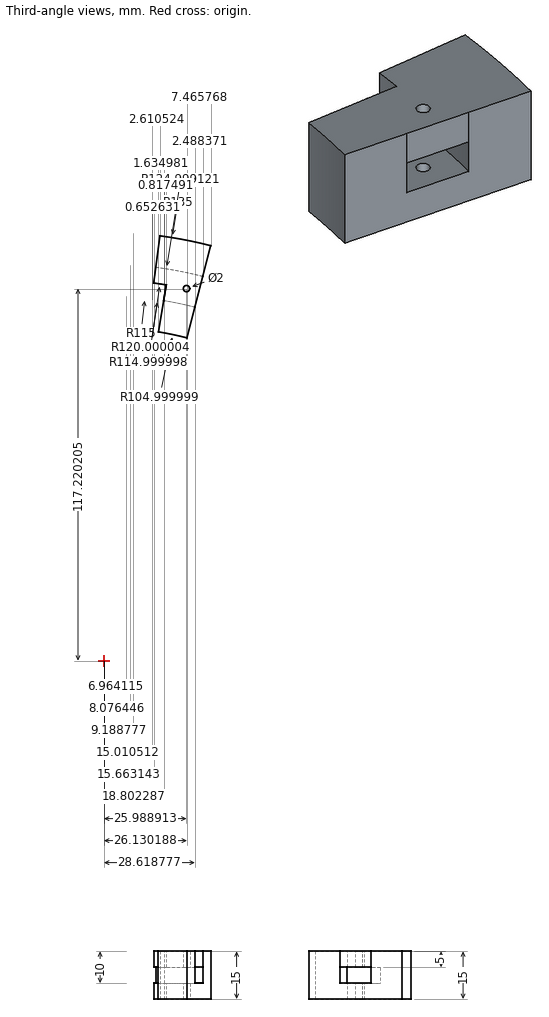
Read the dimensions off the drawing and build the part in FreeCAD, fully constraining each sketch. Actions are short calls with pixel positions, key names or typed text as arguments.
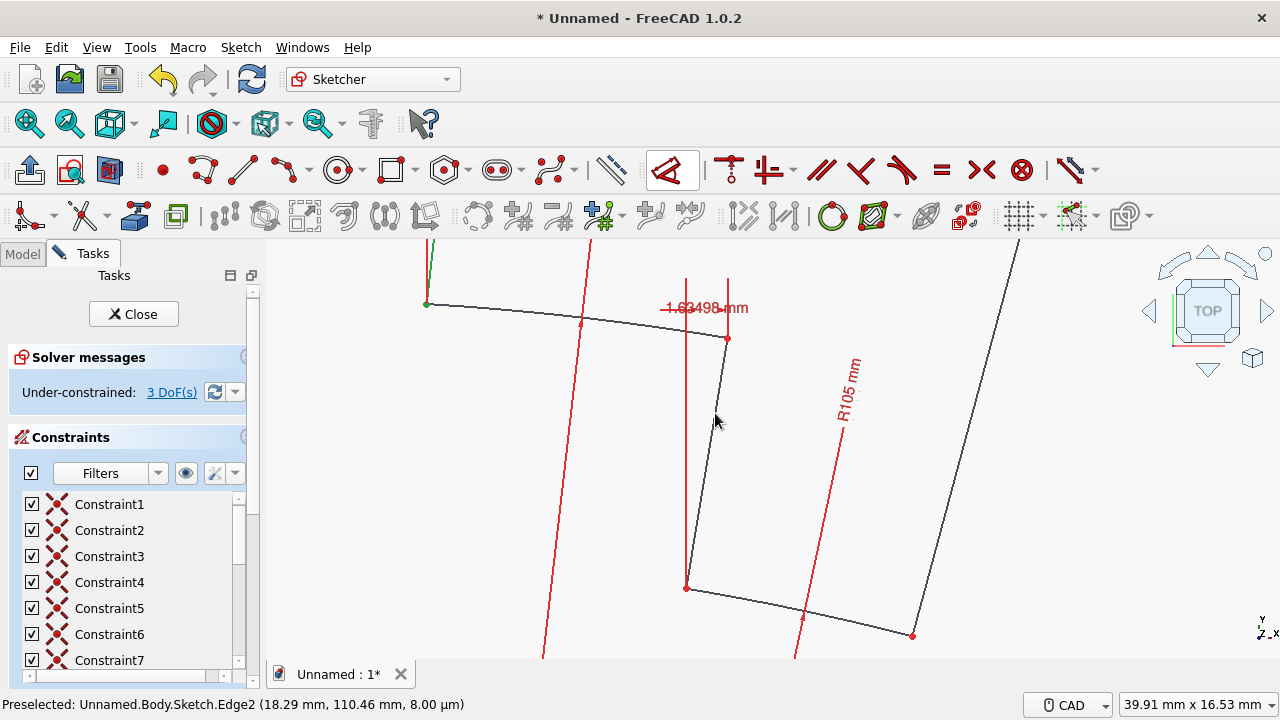
click(972, 416)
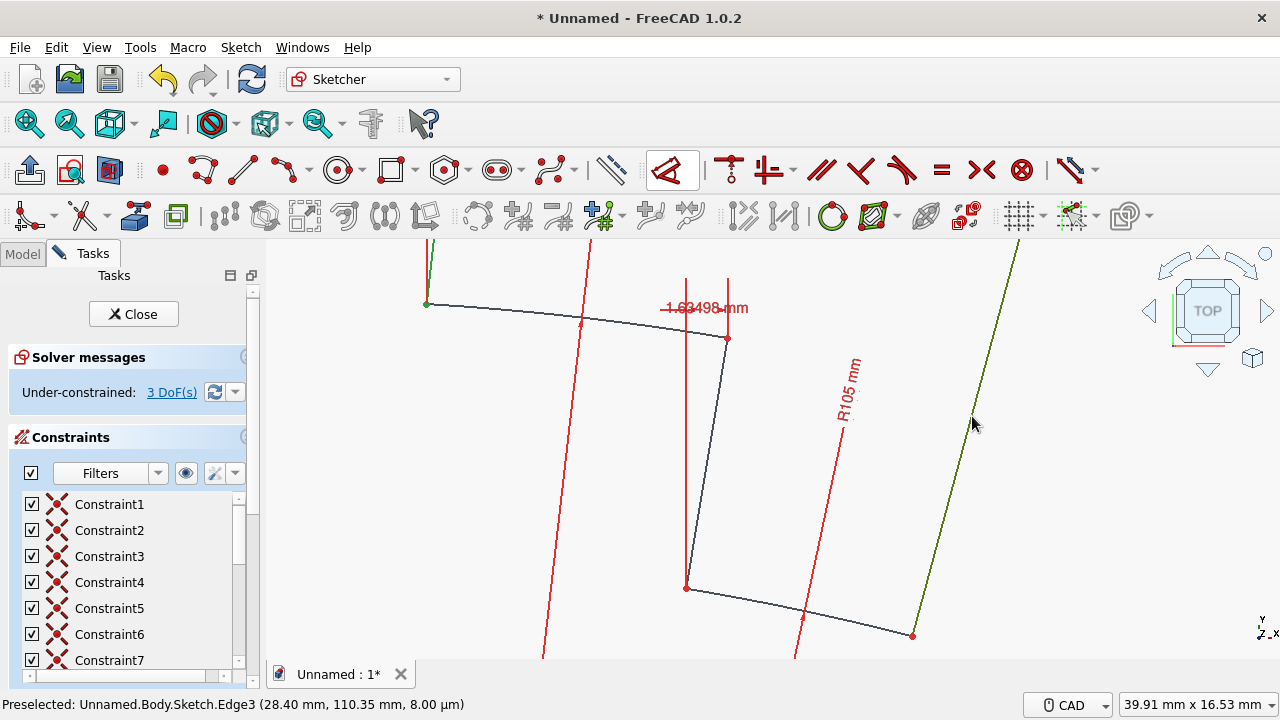
key(l)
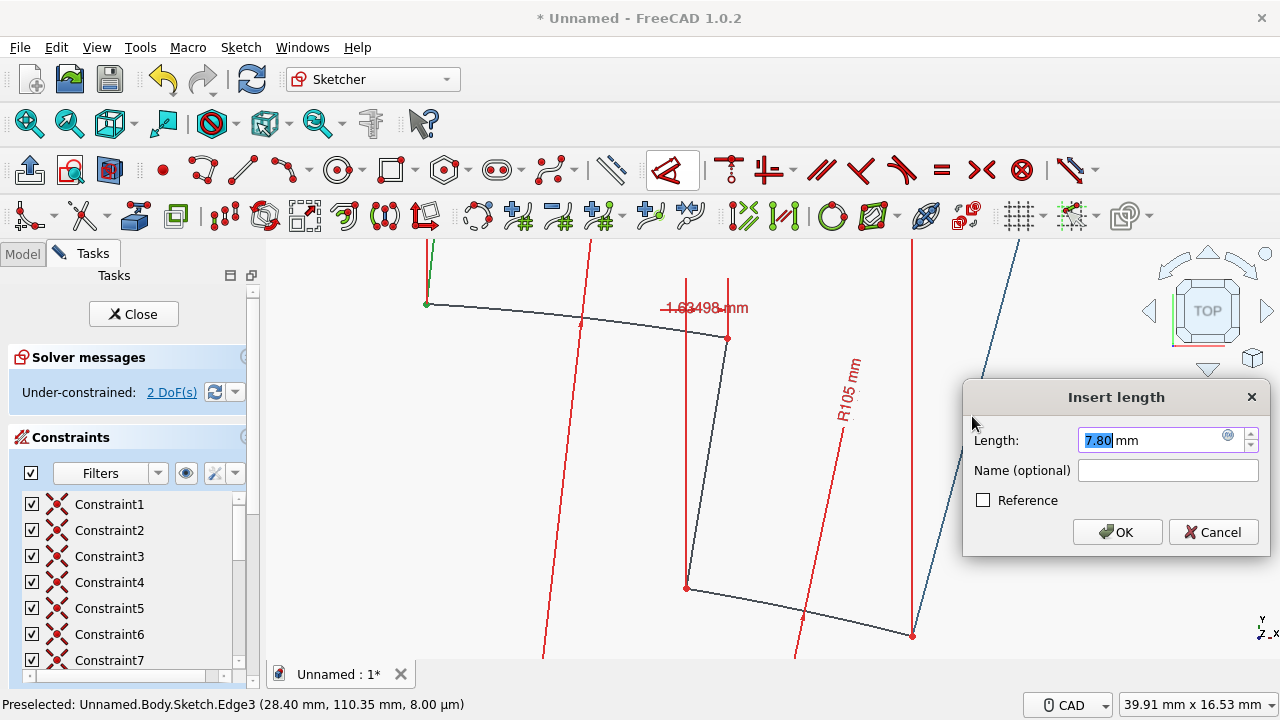
text(7.465768)
key(Return)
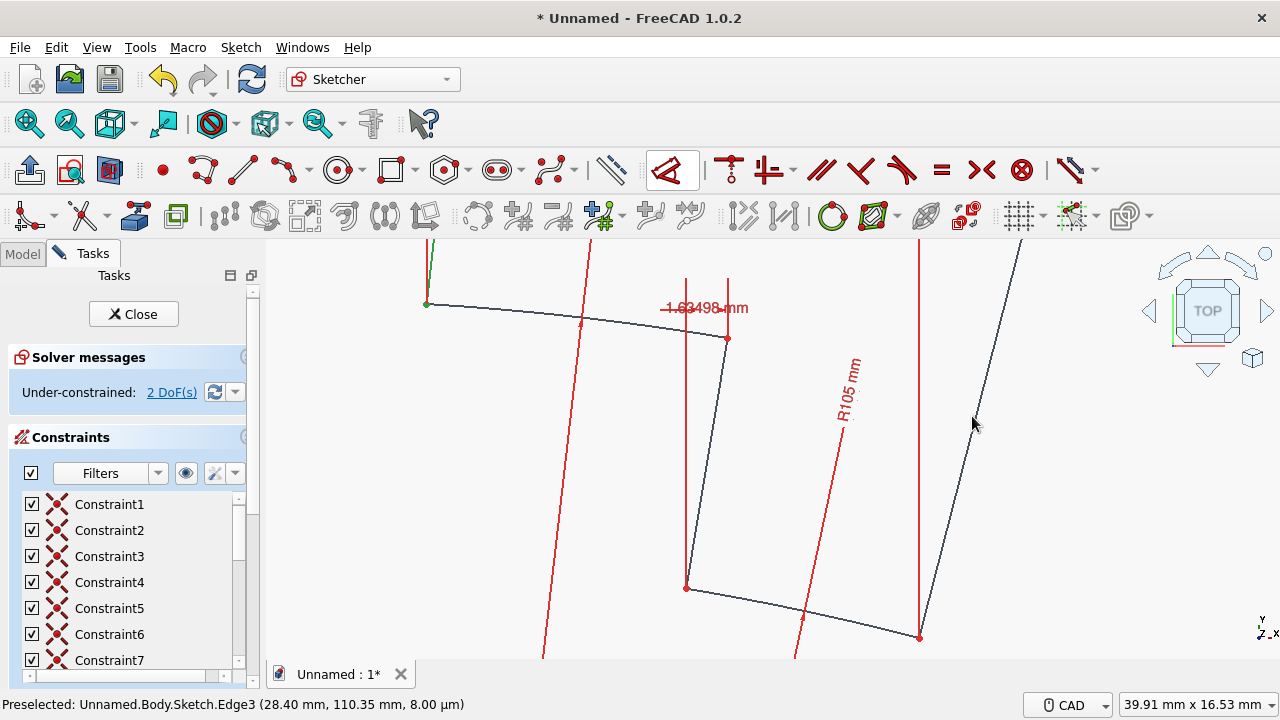
click(728, 338)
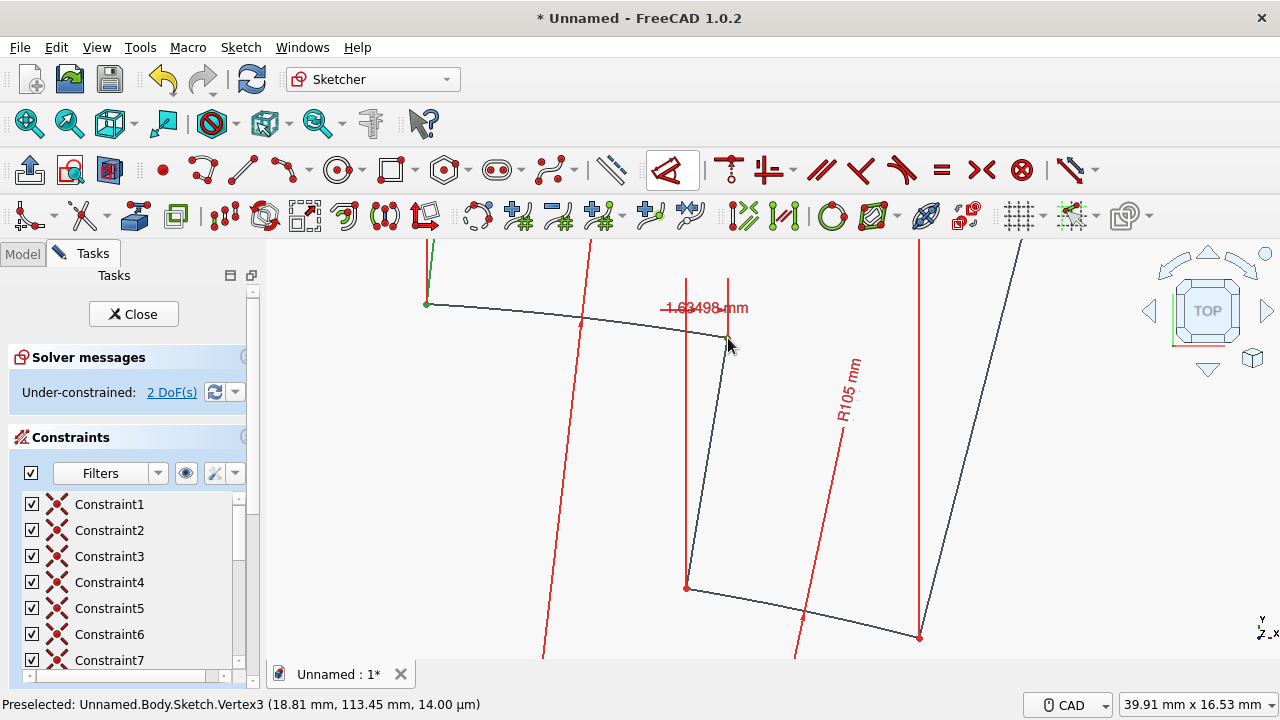
click(694, 170)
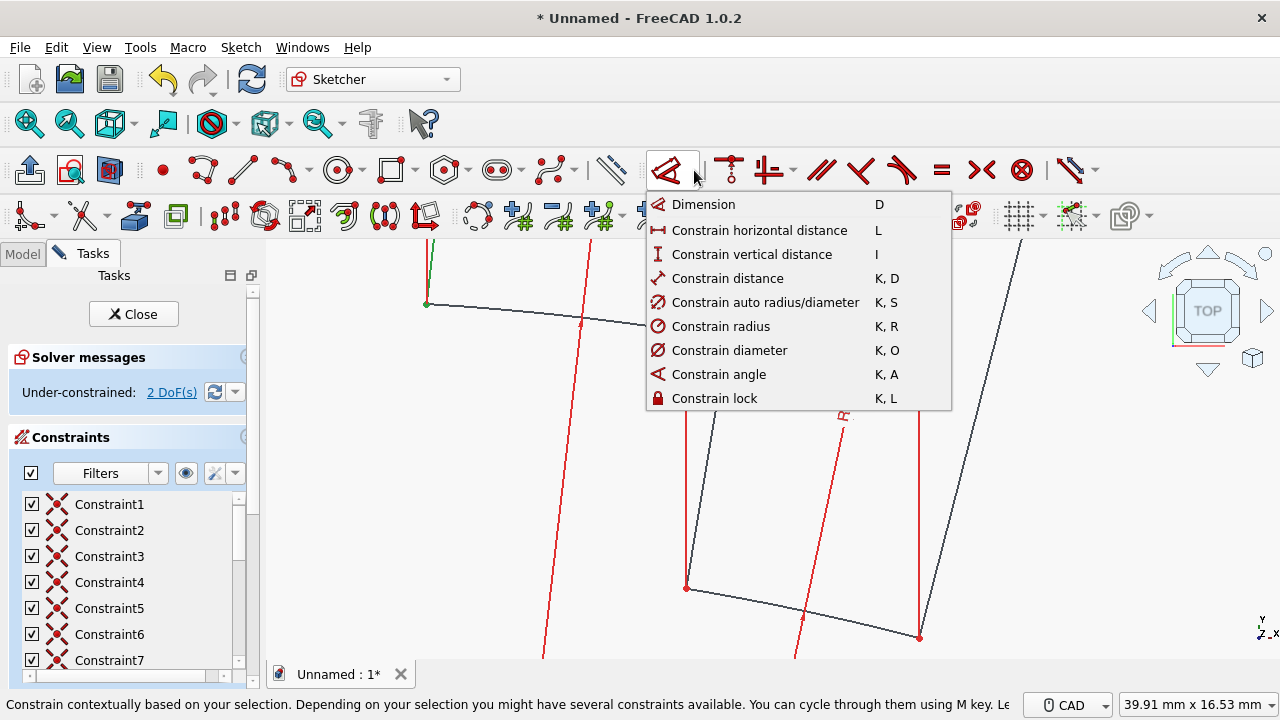
click(799, 230)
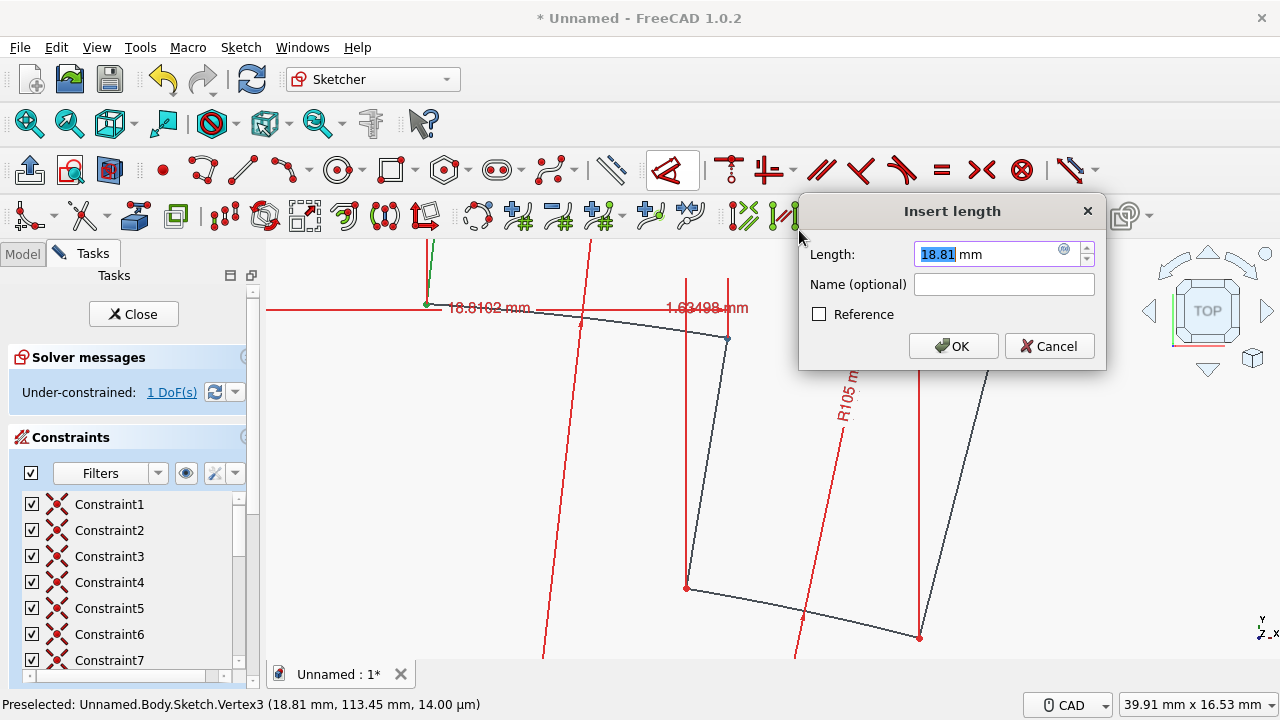
text(18.802287)
key(Return)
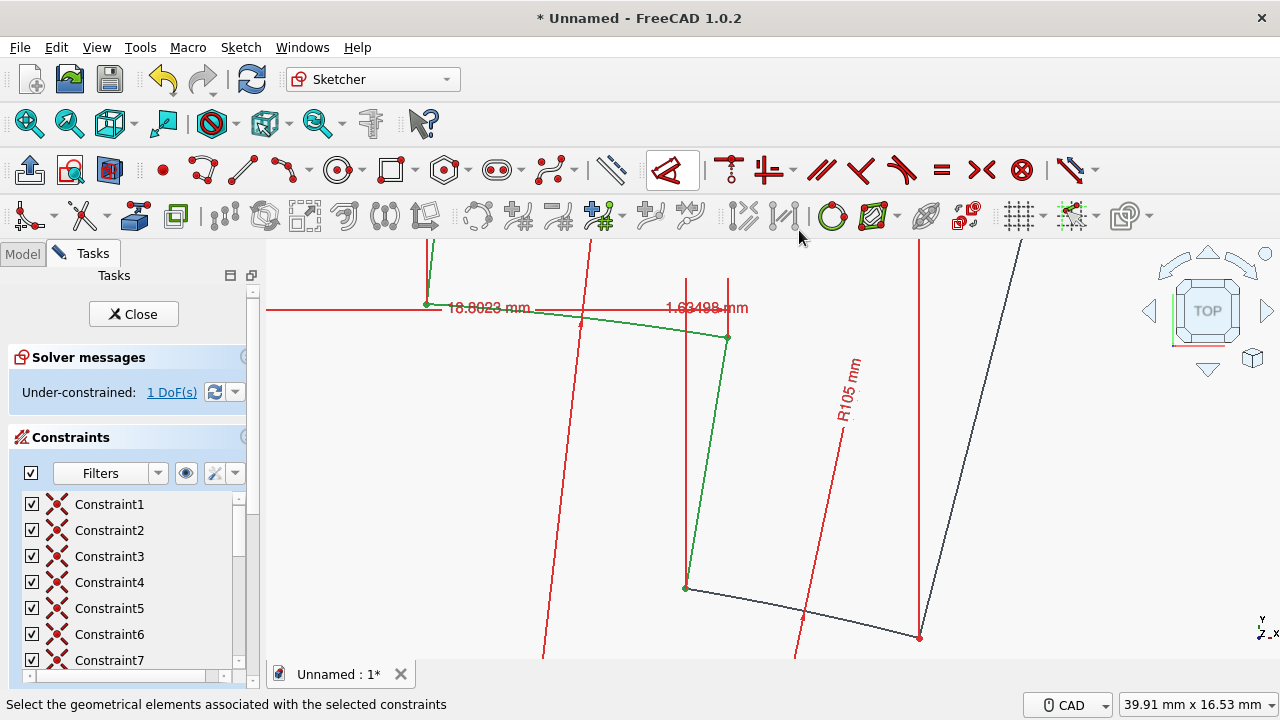
scroll(678, 549, down, 6)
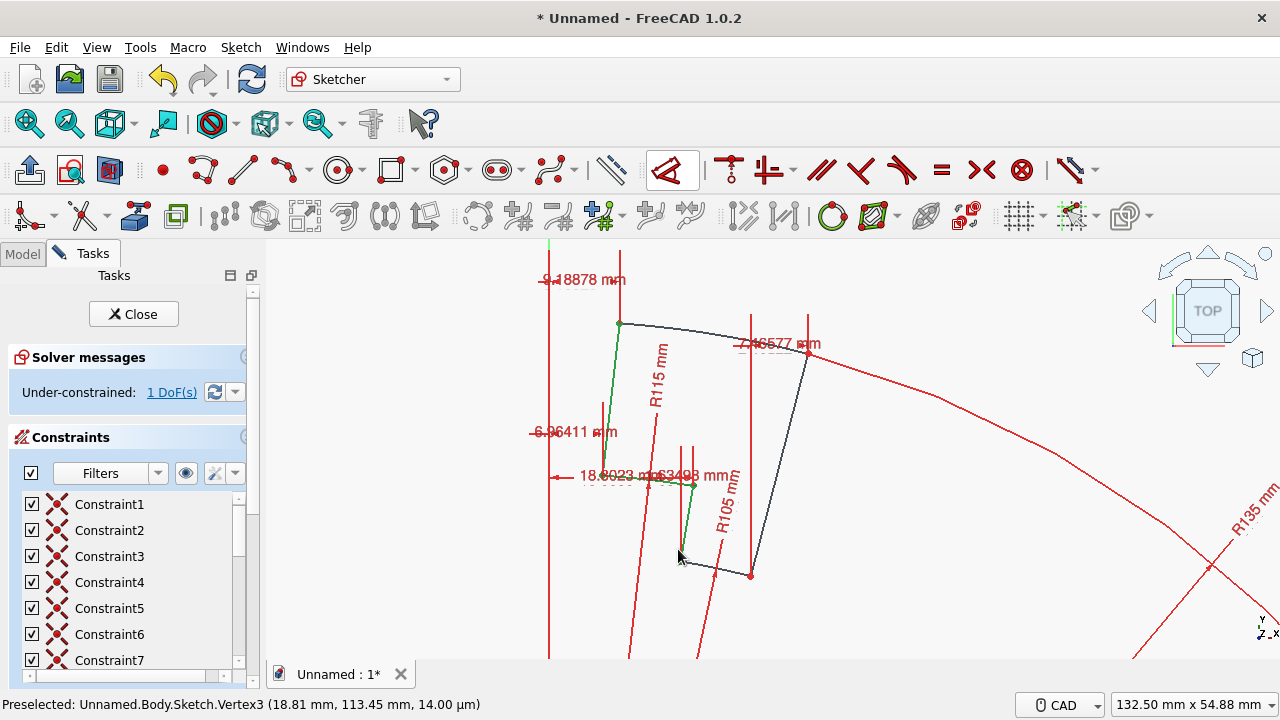
click(751, 576)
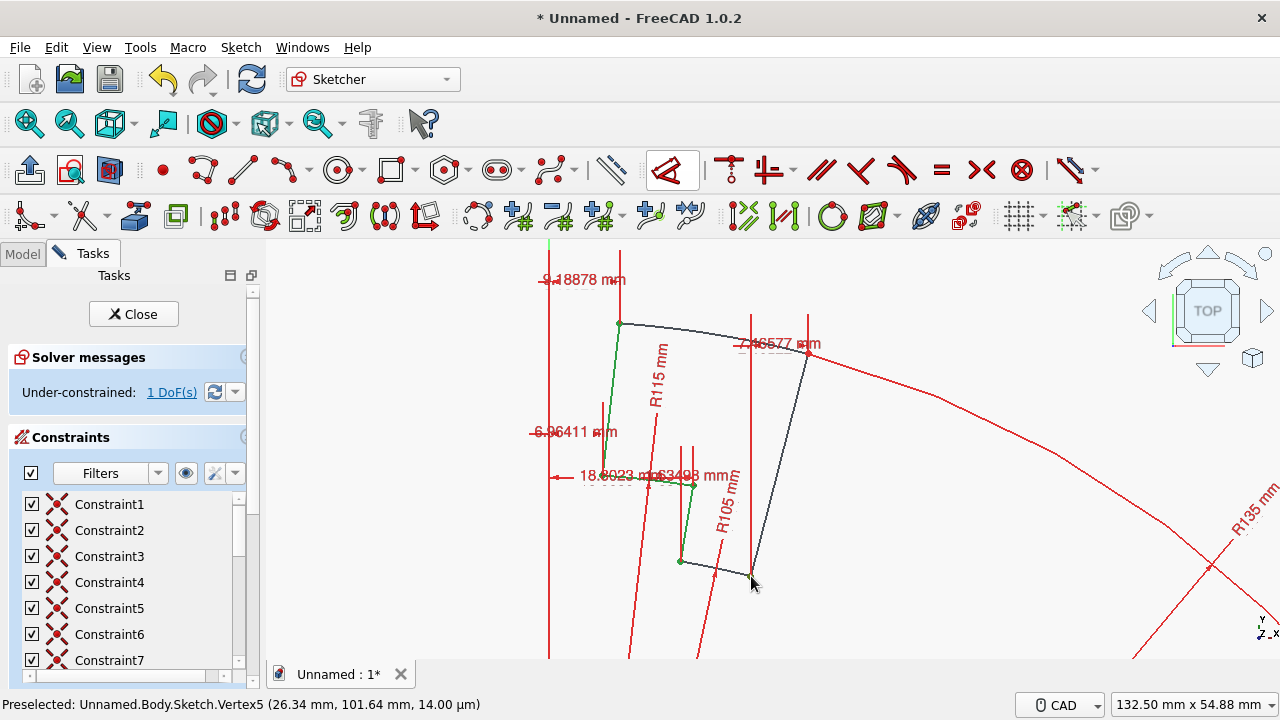
key(l)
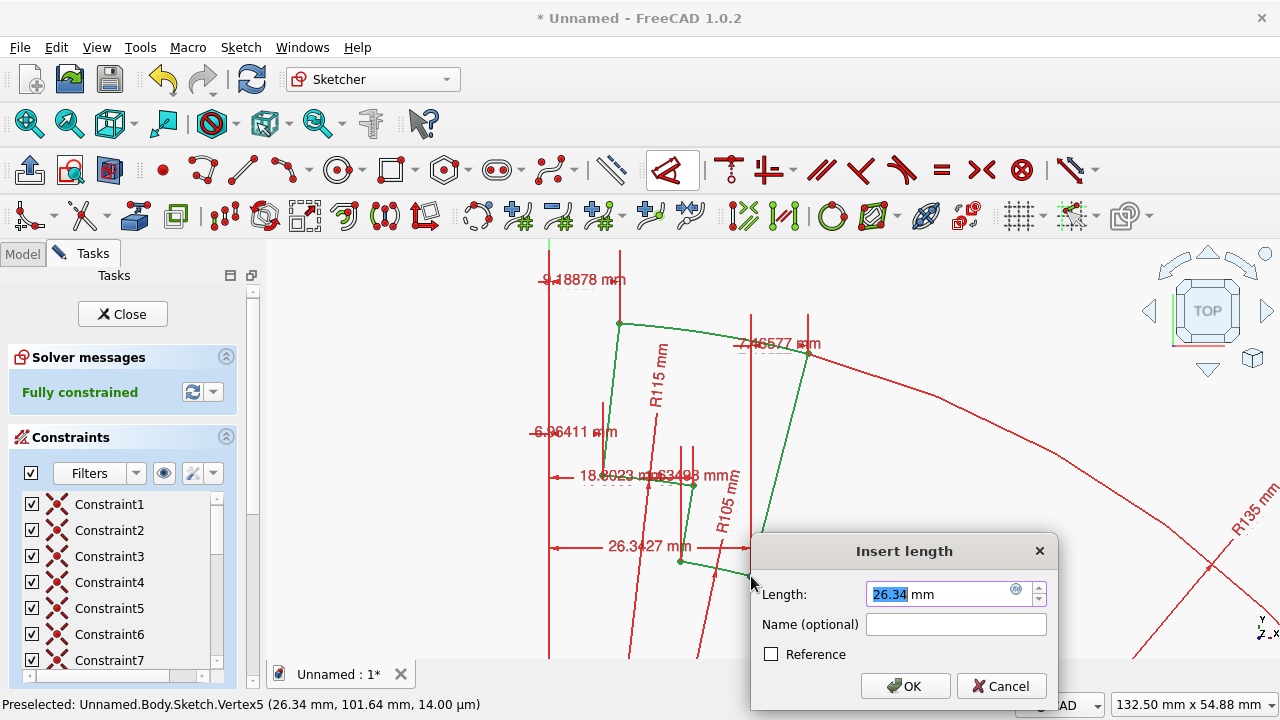
text(26.130188)
key(Return)